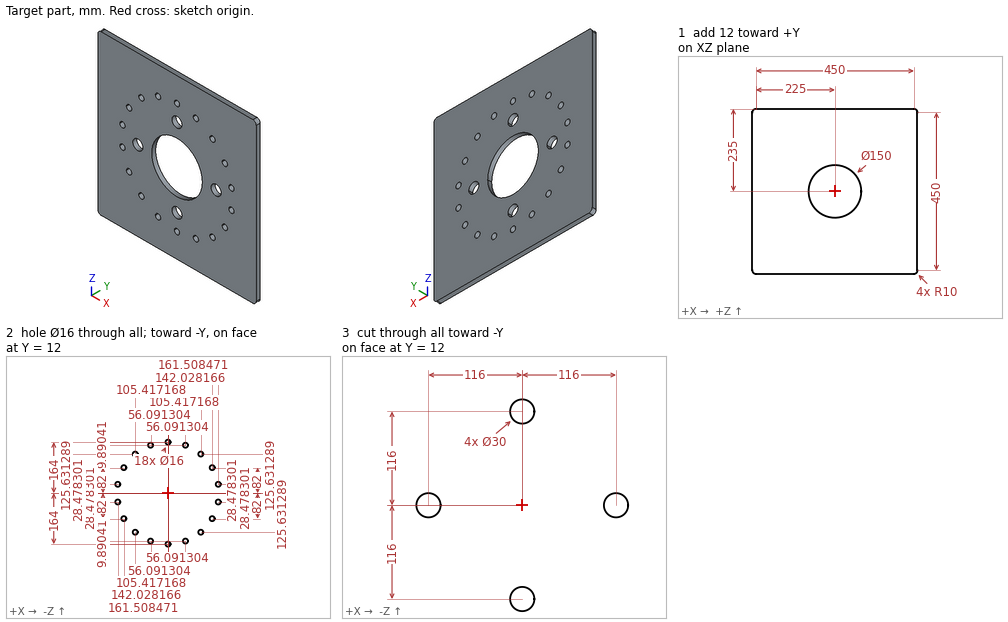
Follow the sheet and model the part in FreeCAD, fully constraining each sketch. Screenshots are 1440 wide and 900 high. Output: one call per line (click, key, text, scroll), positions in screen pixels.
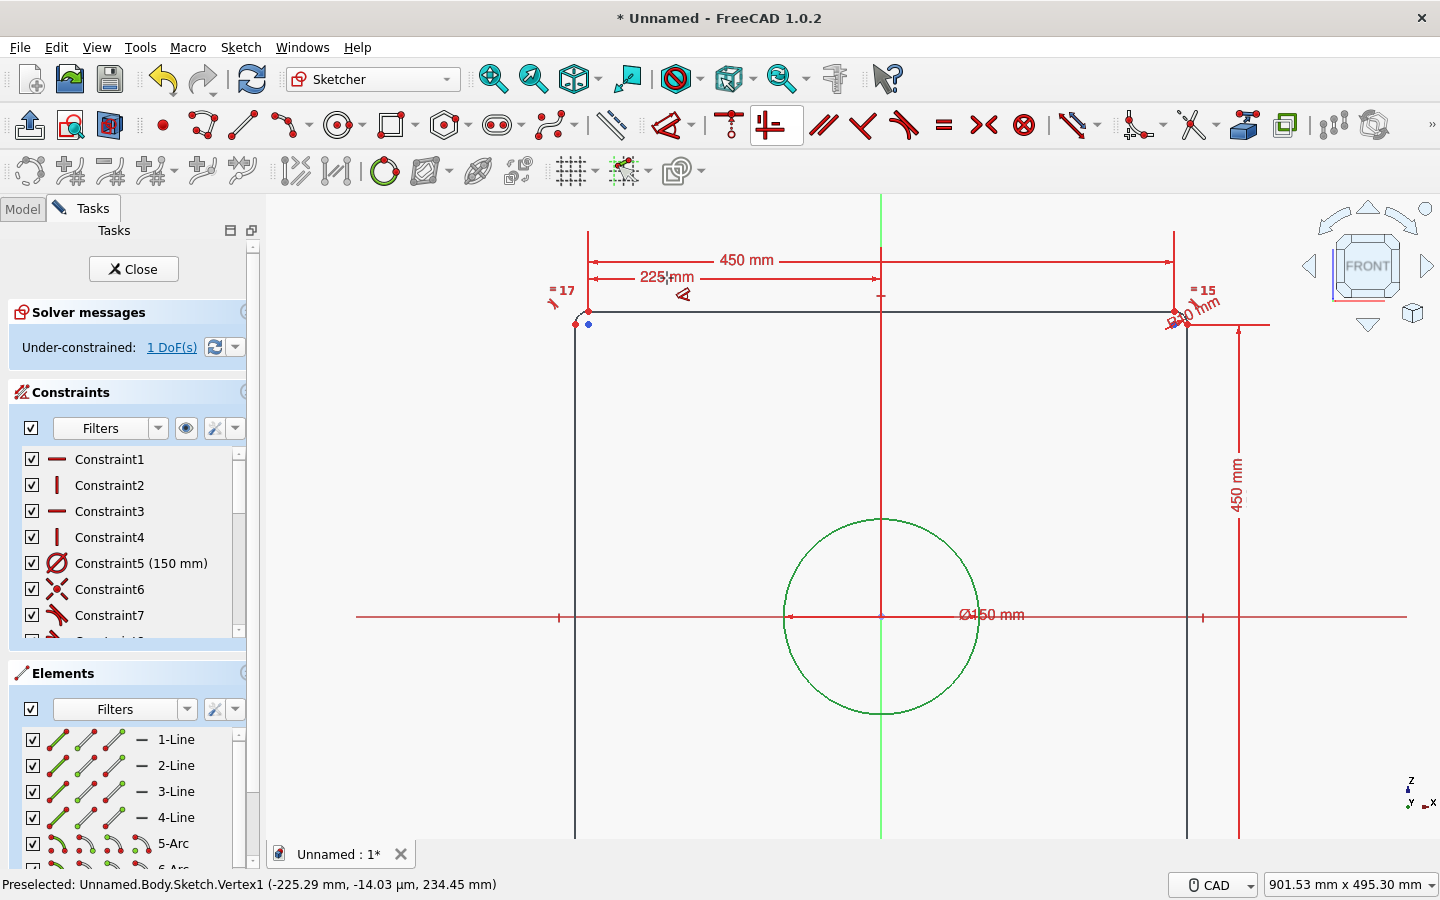
click(588, 312)
click(554, 464)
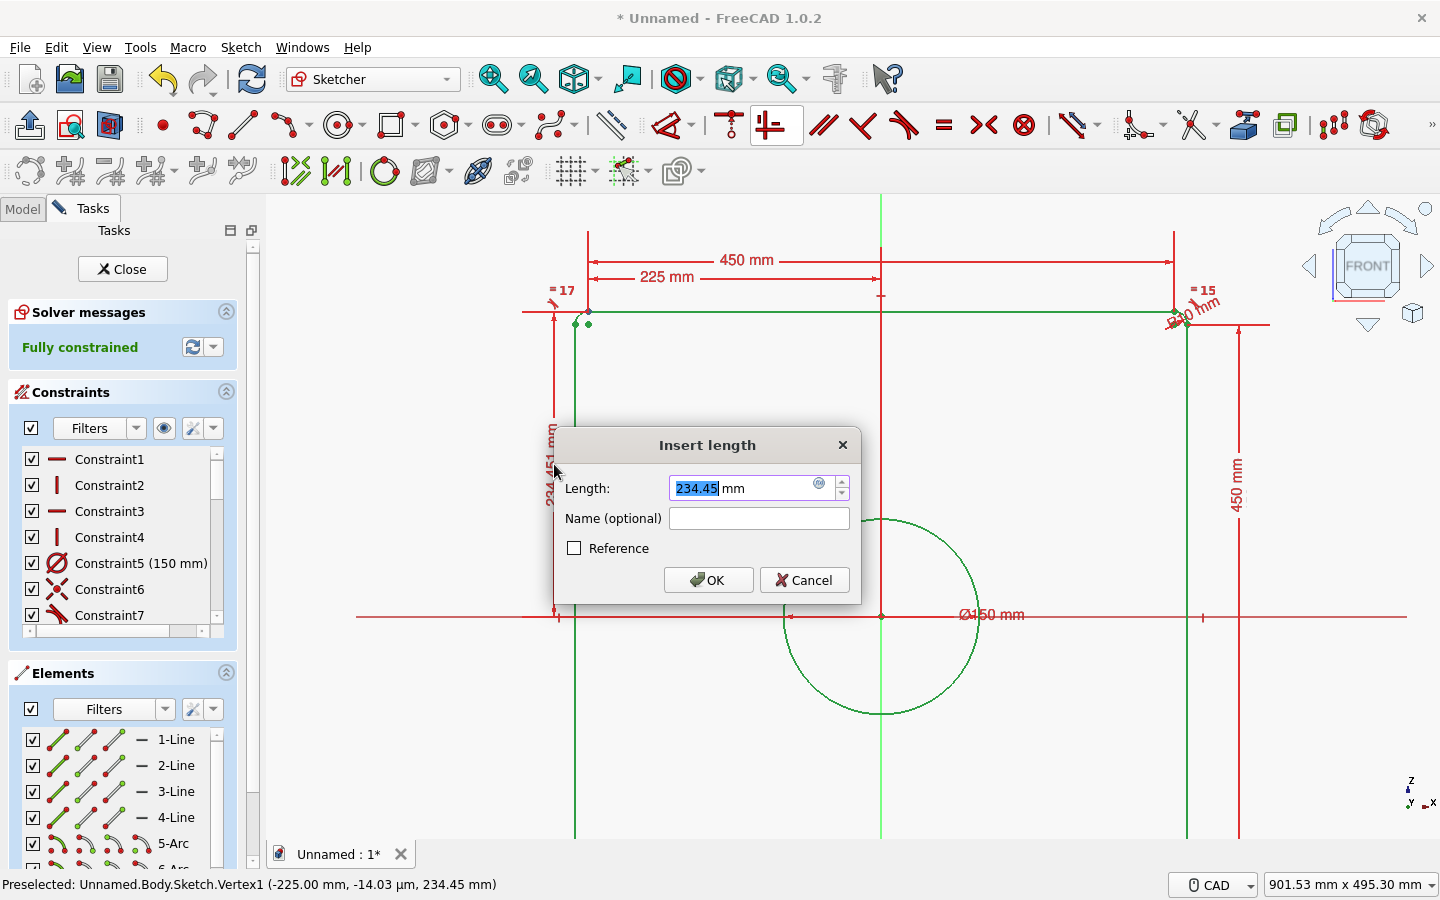
text(235)
key(Return)
key(Escape)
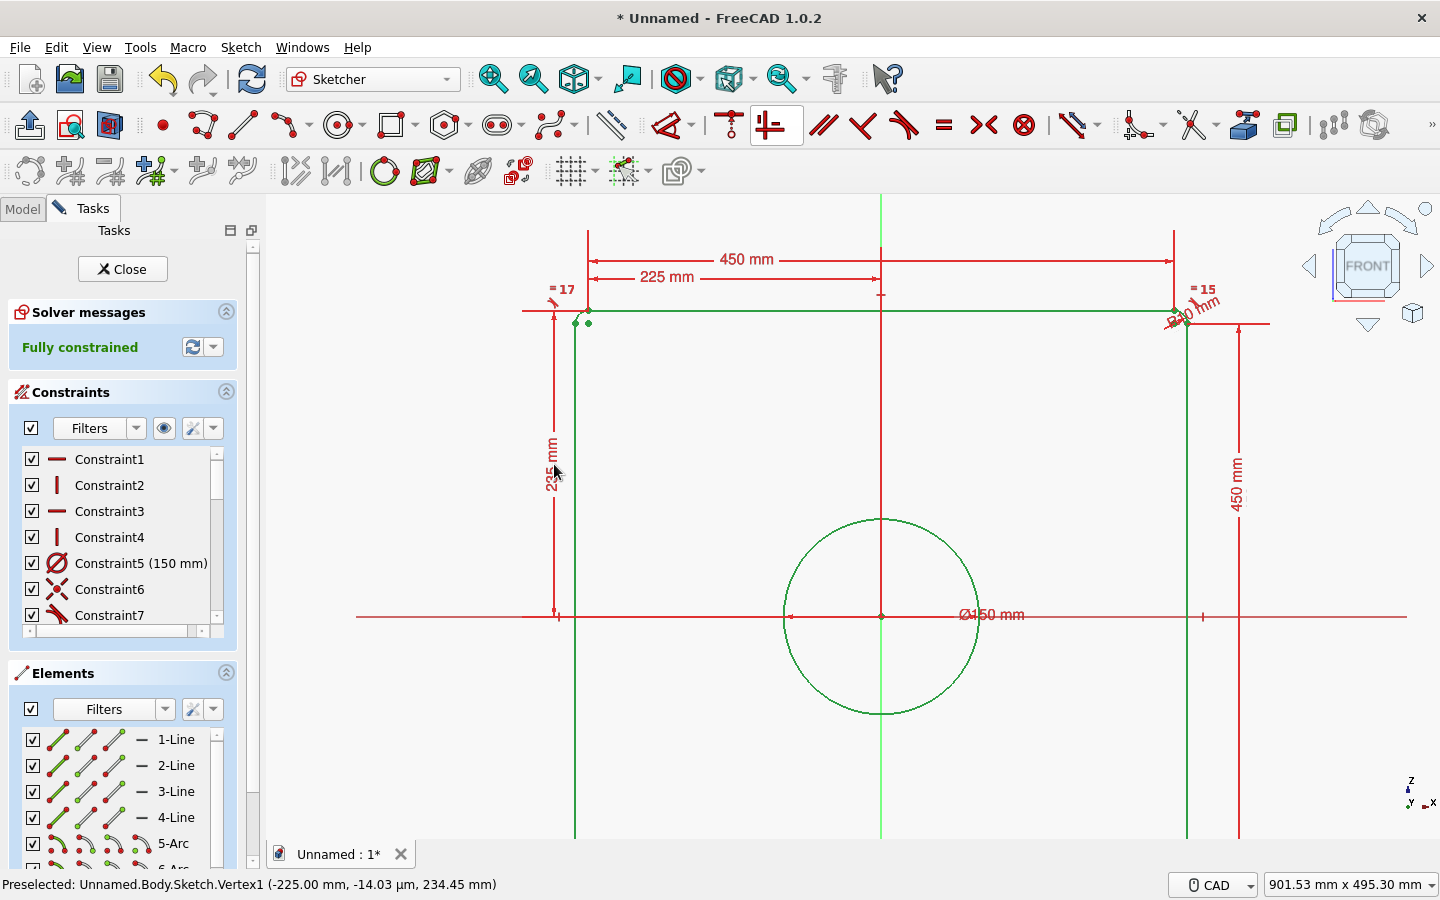
click(123, 269)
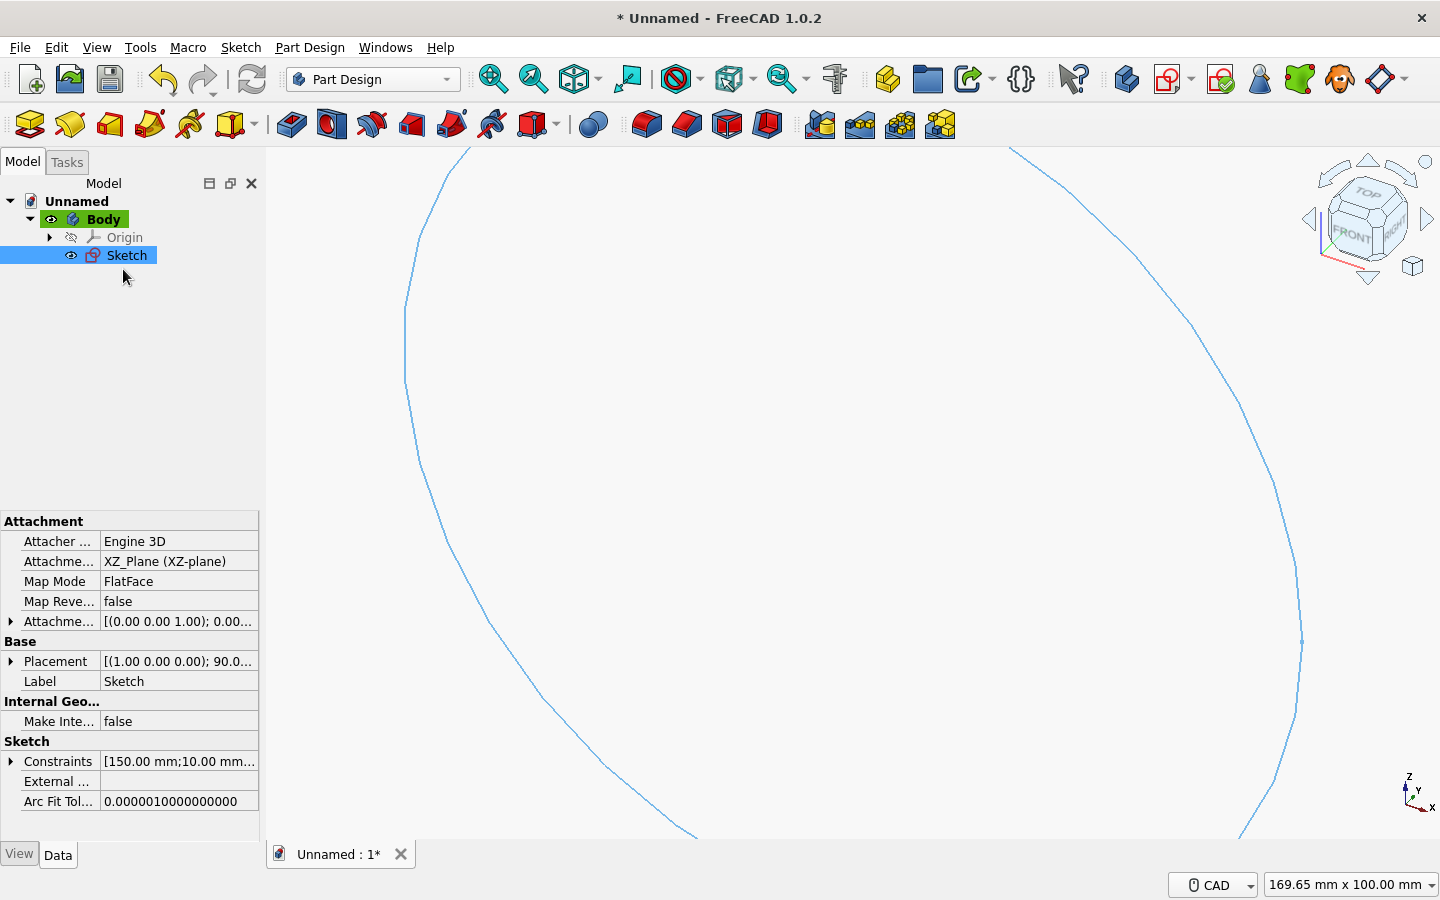
click(30, 124)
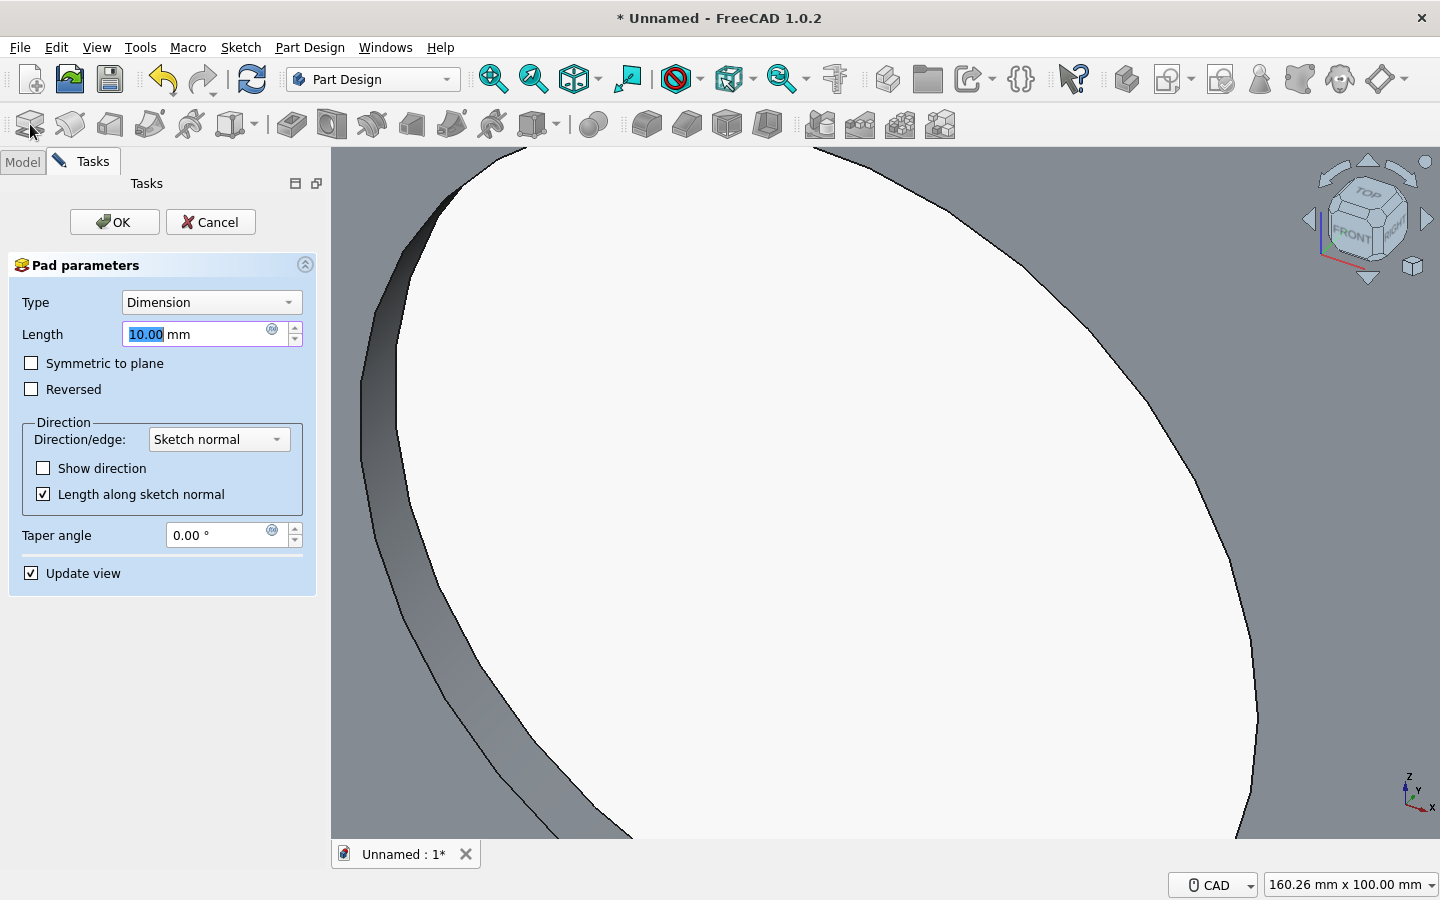
text(12)
key(Tab)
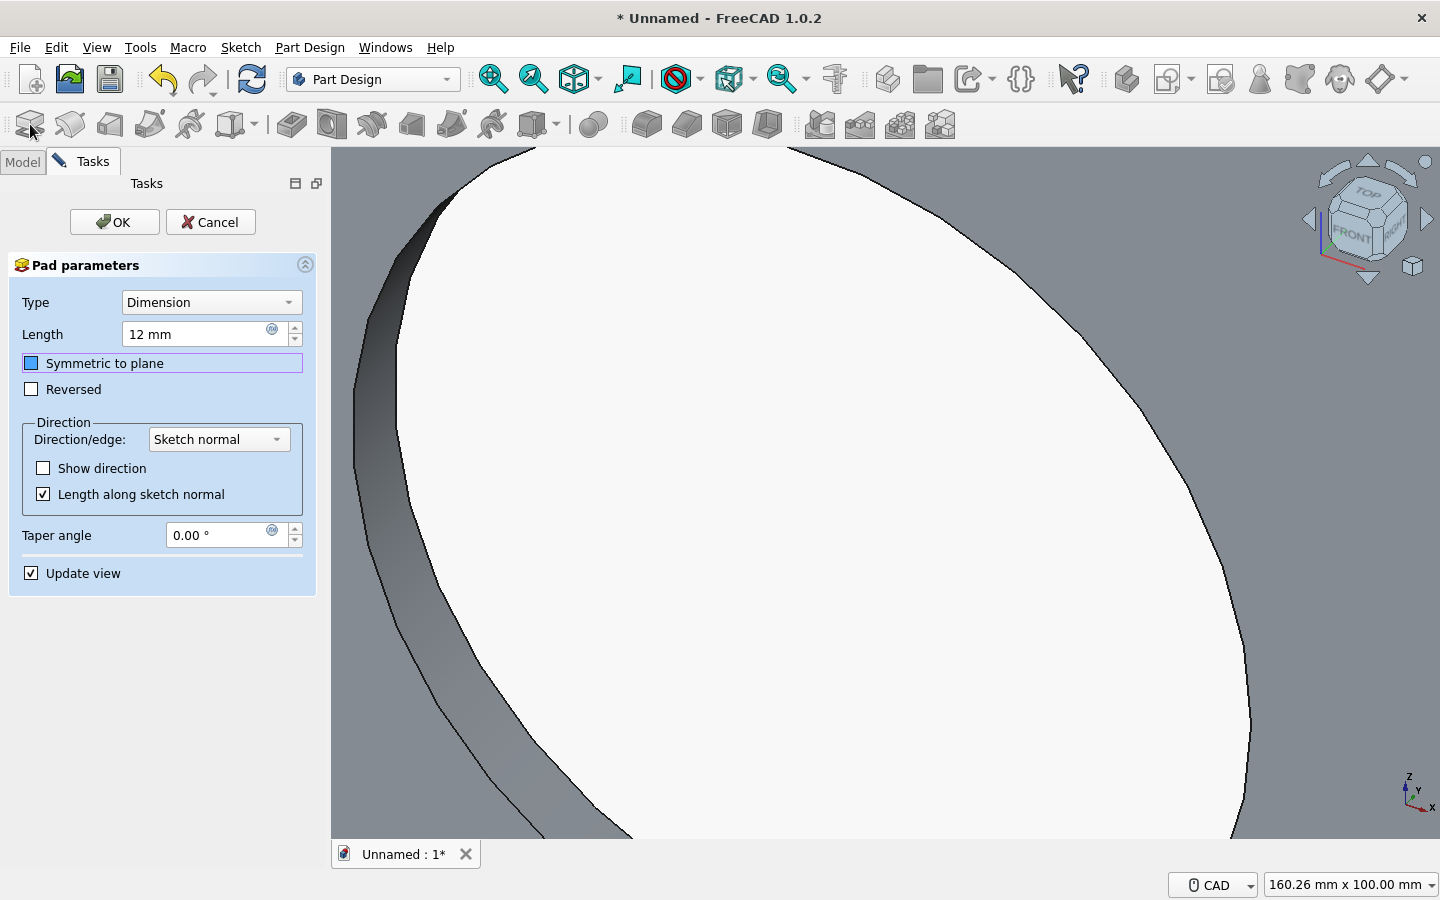
click(30, 389)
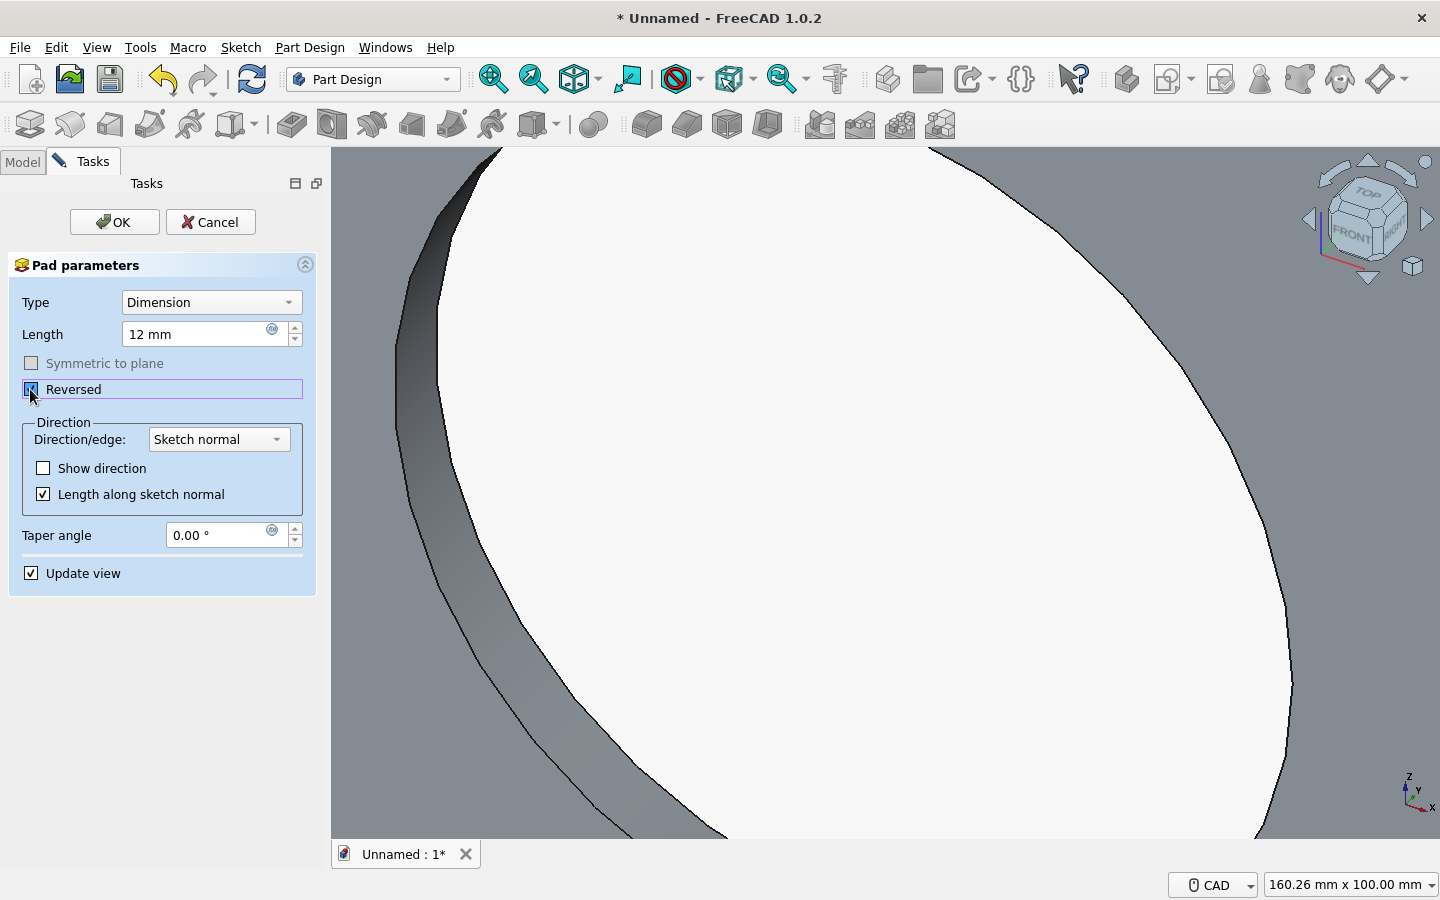
click(115, 222)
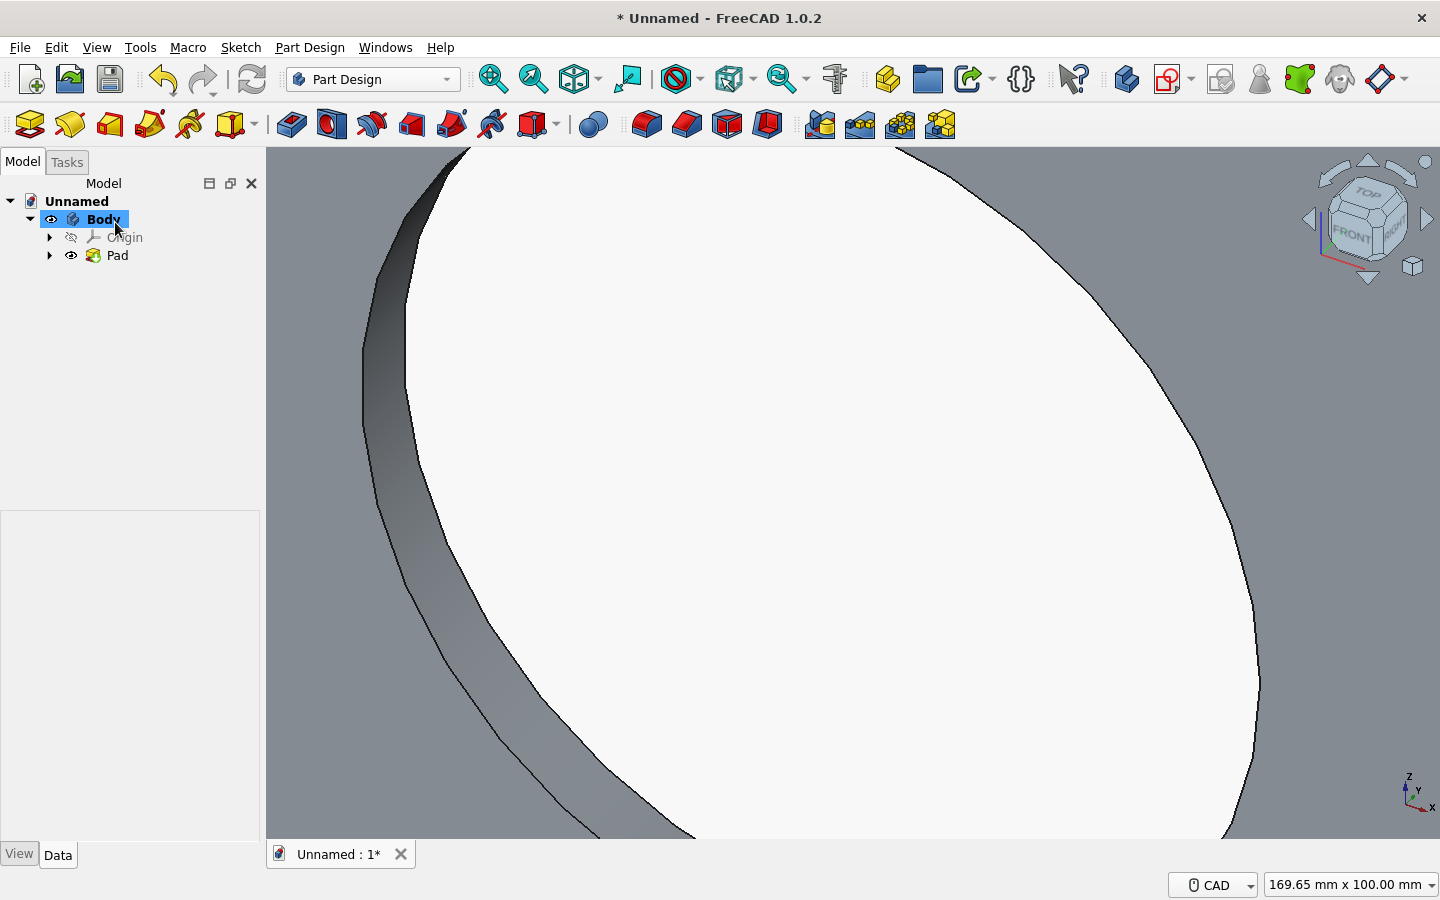
click(494, 80)